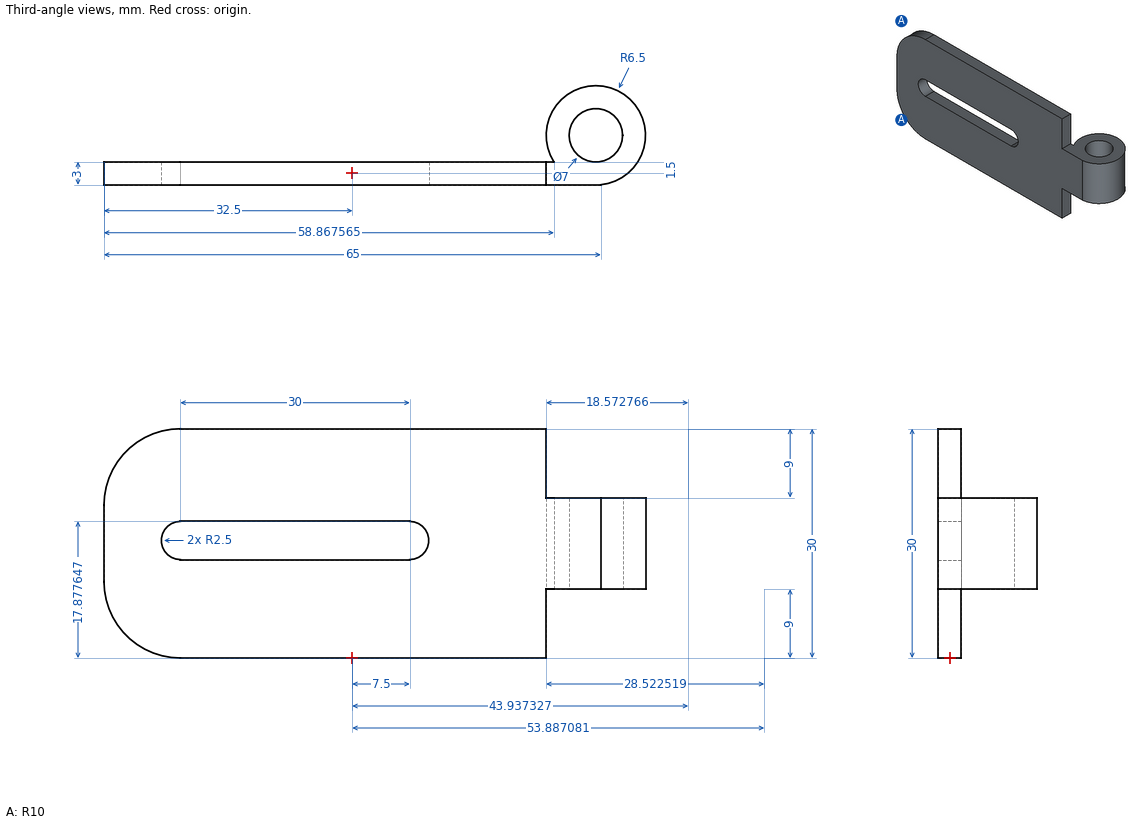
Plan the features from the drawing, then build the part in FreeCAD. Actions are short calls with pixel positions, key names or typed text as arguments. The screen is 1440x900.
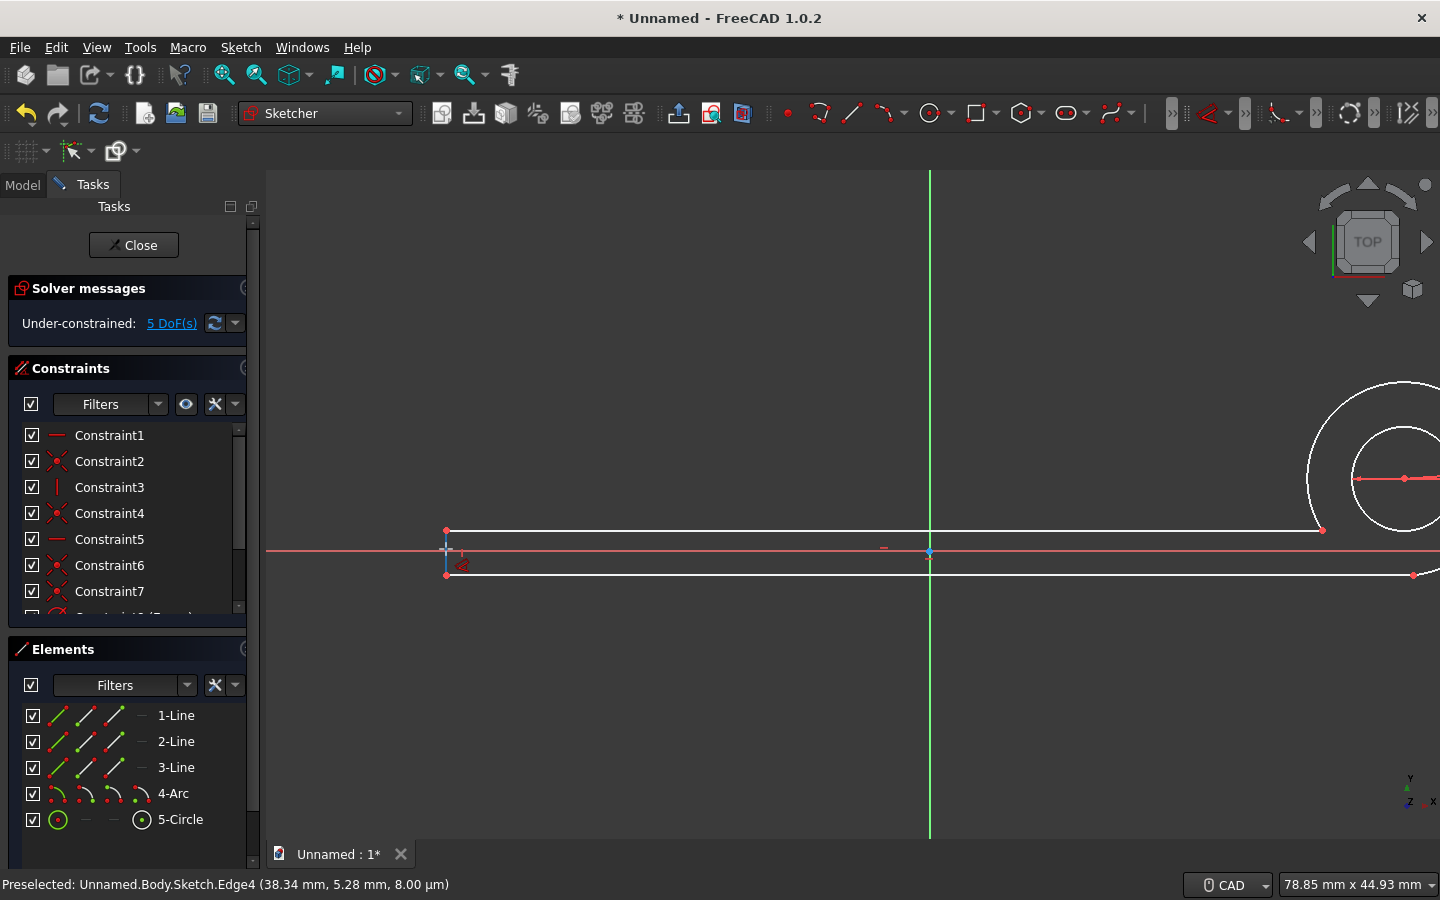
click(446, 549)
click(412, 537)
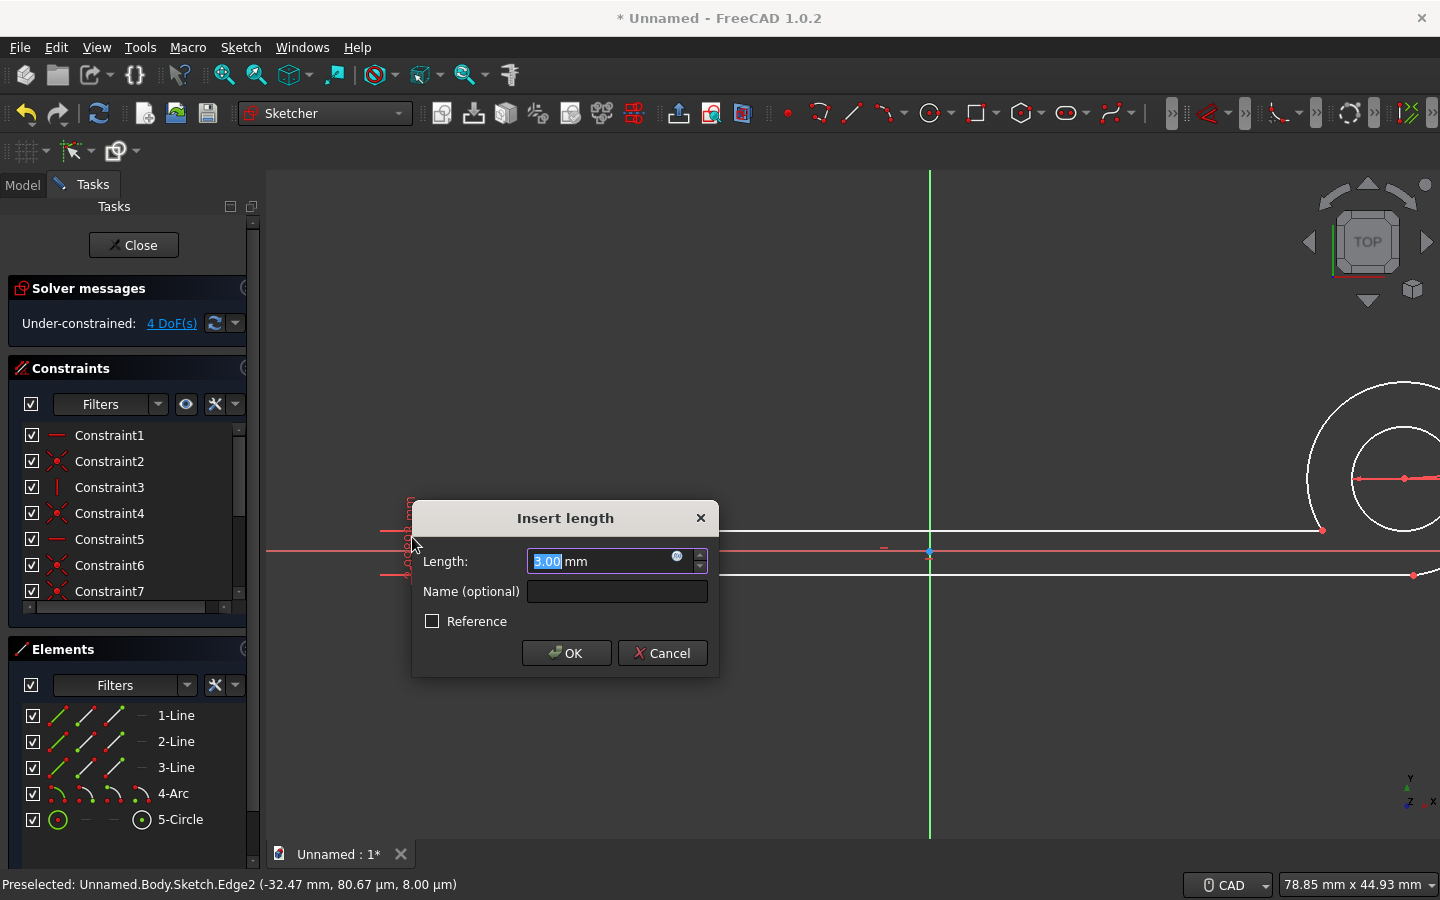
text(3)
key(Return)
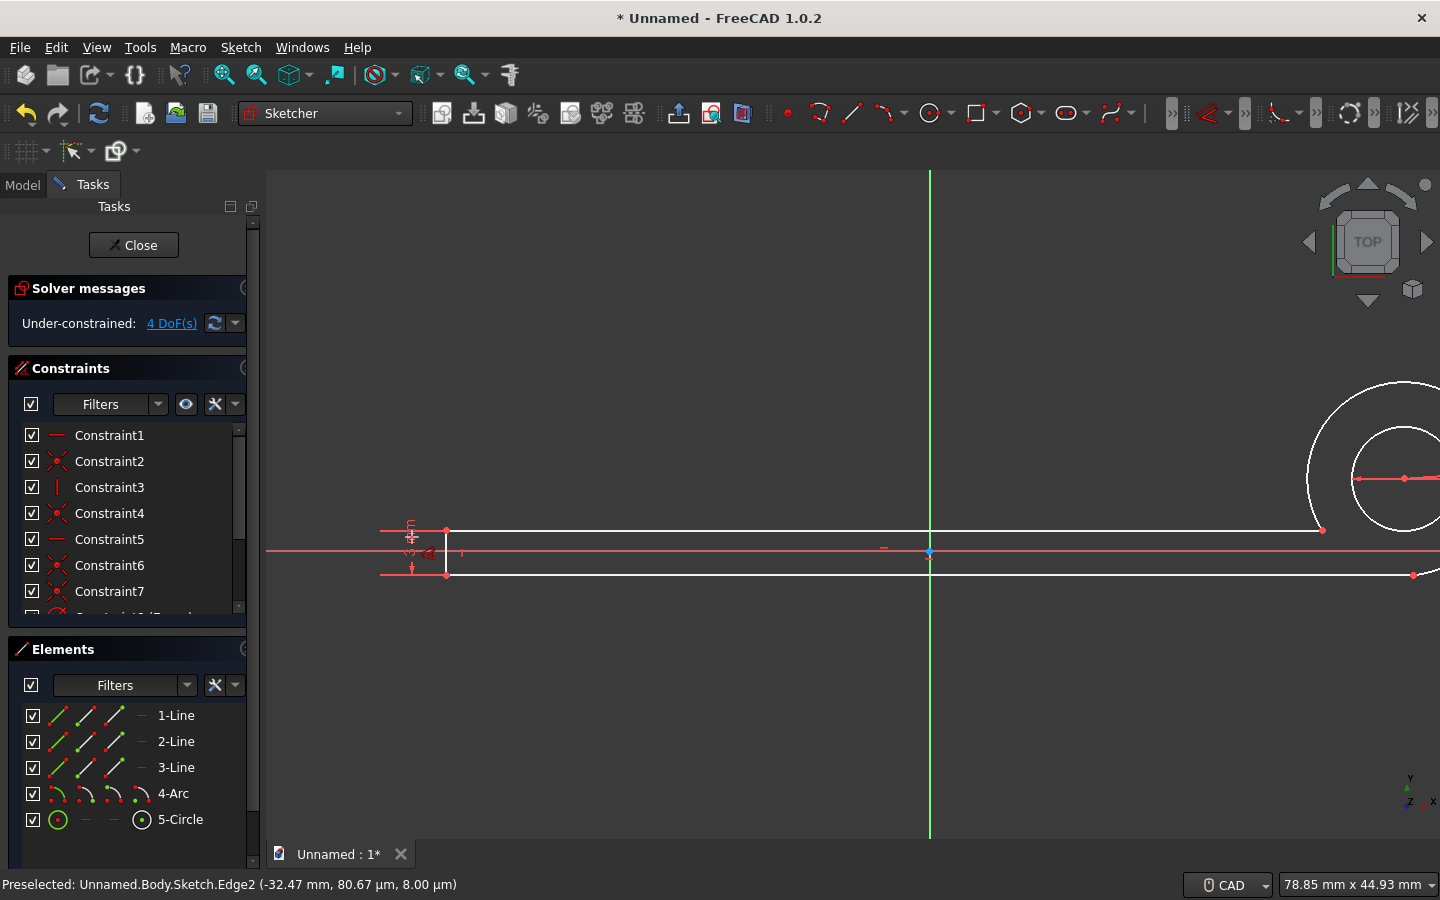
click(736, 575)
click(861, 609)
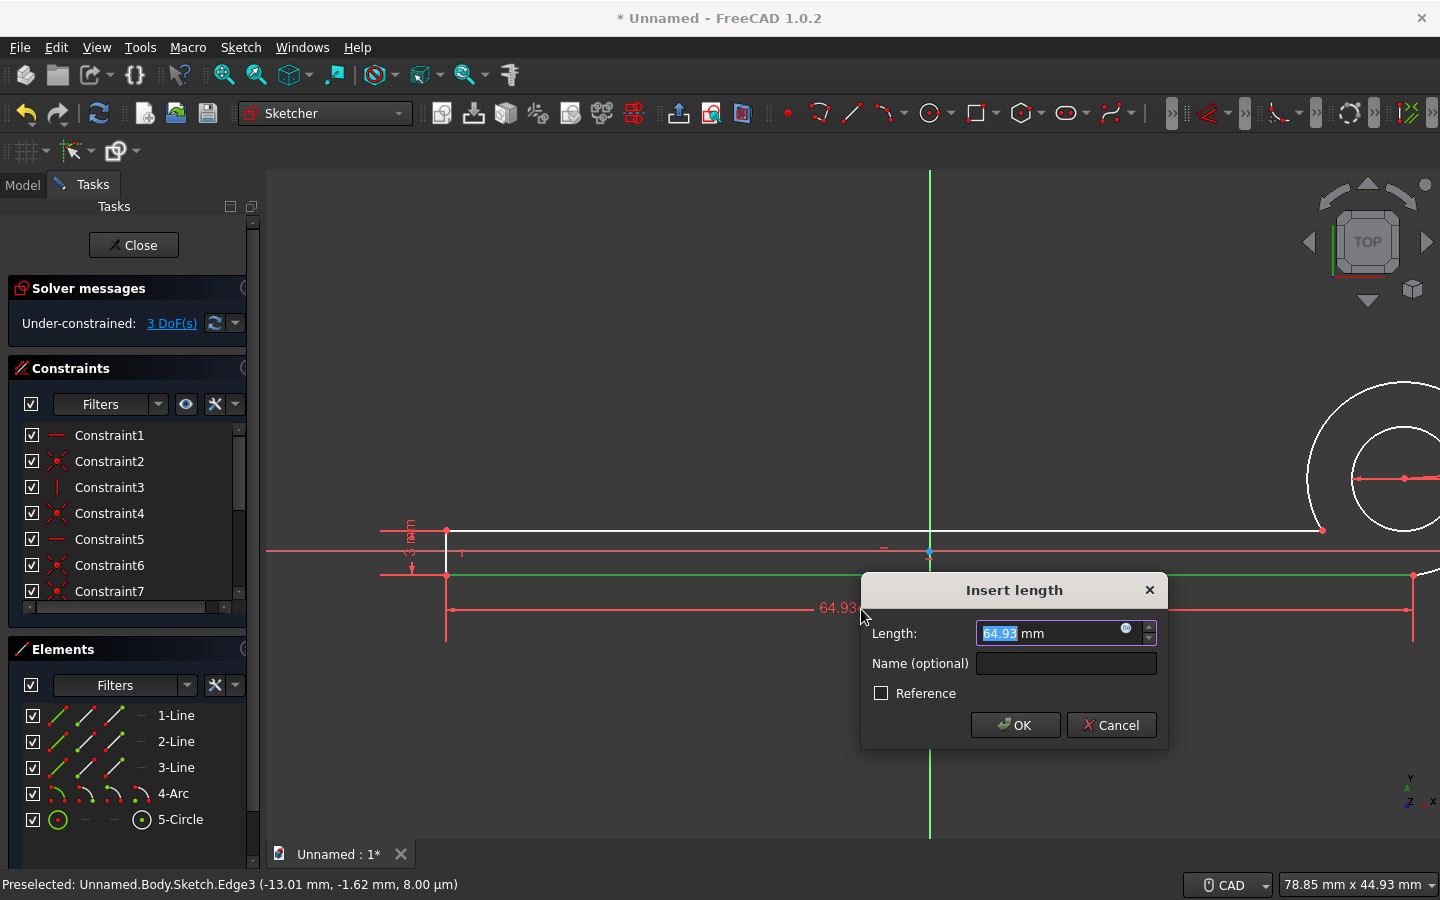
text(65)
key(Return)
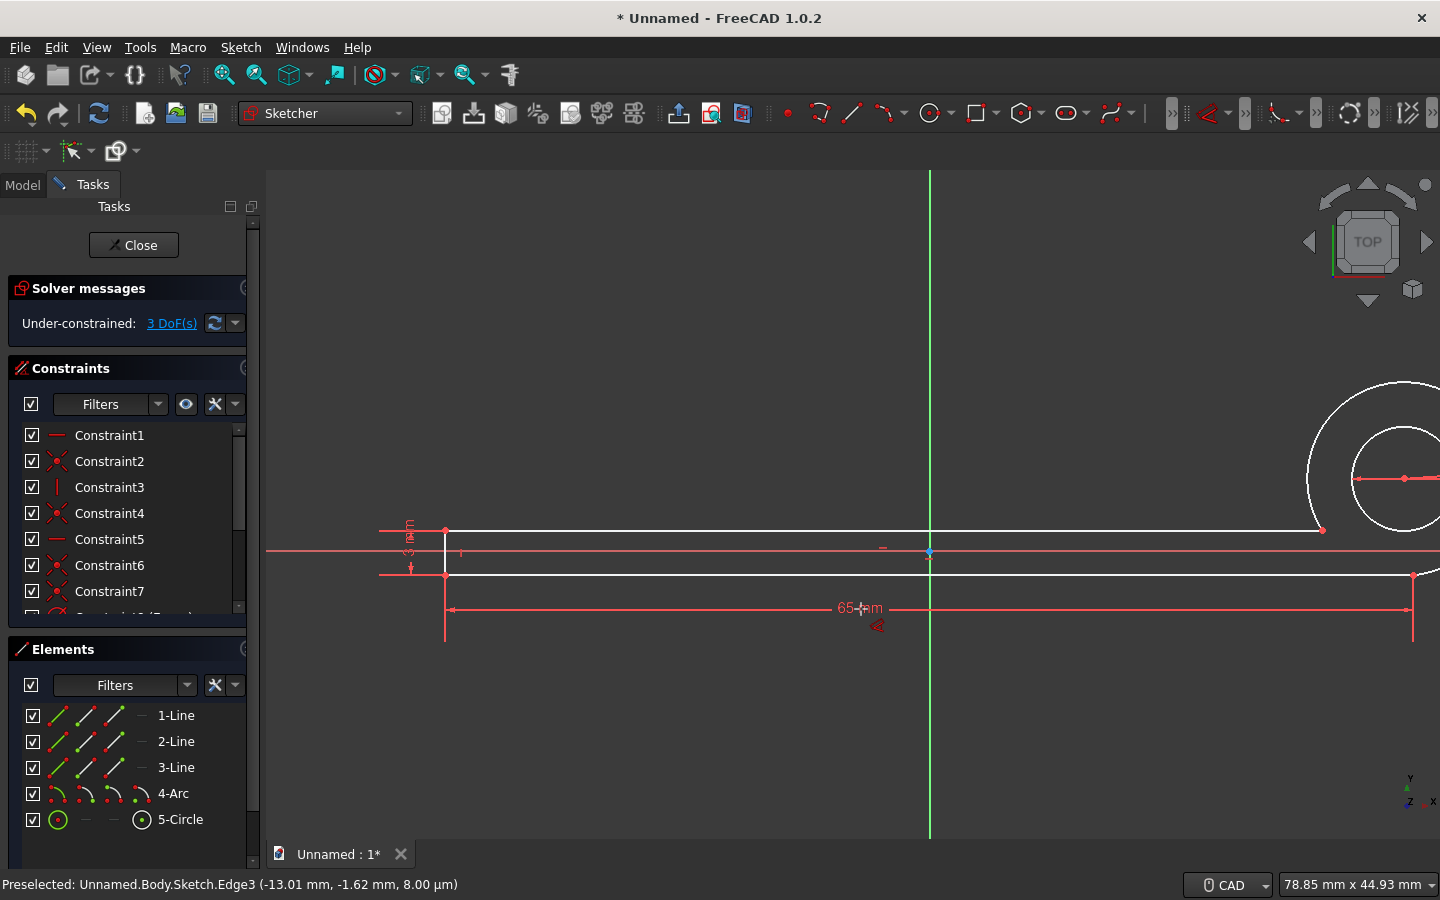
scroll(446, 550, down, 2)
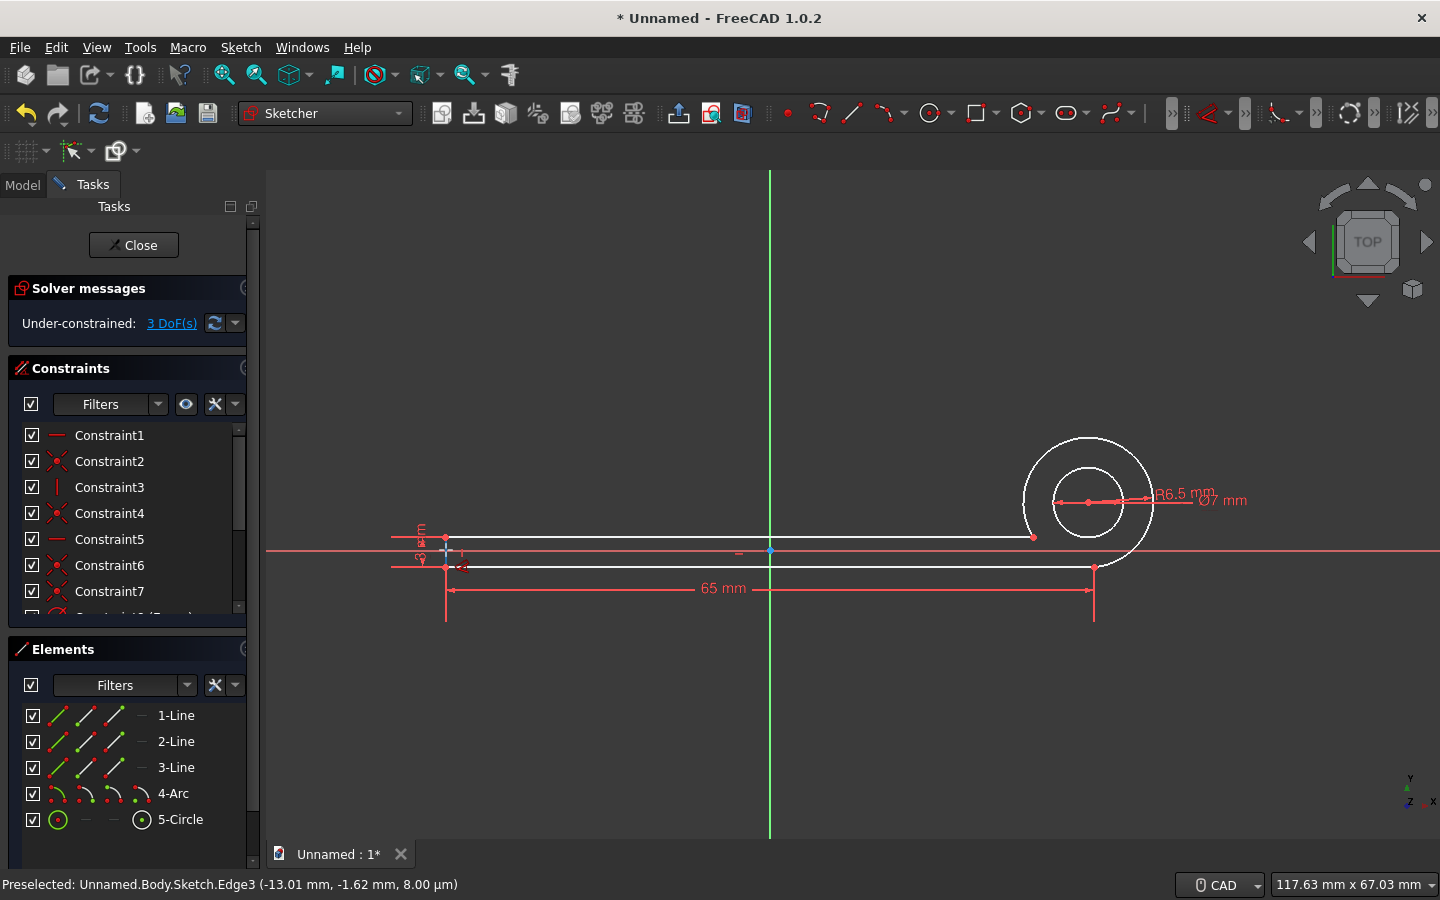
scroll(1033, 537, up, 5)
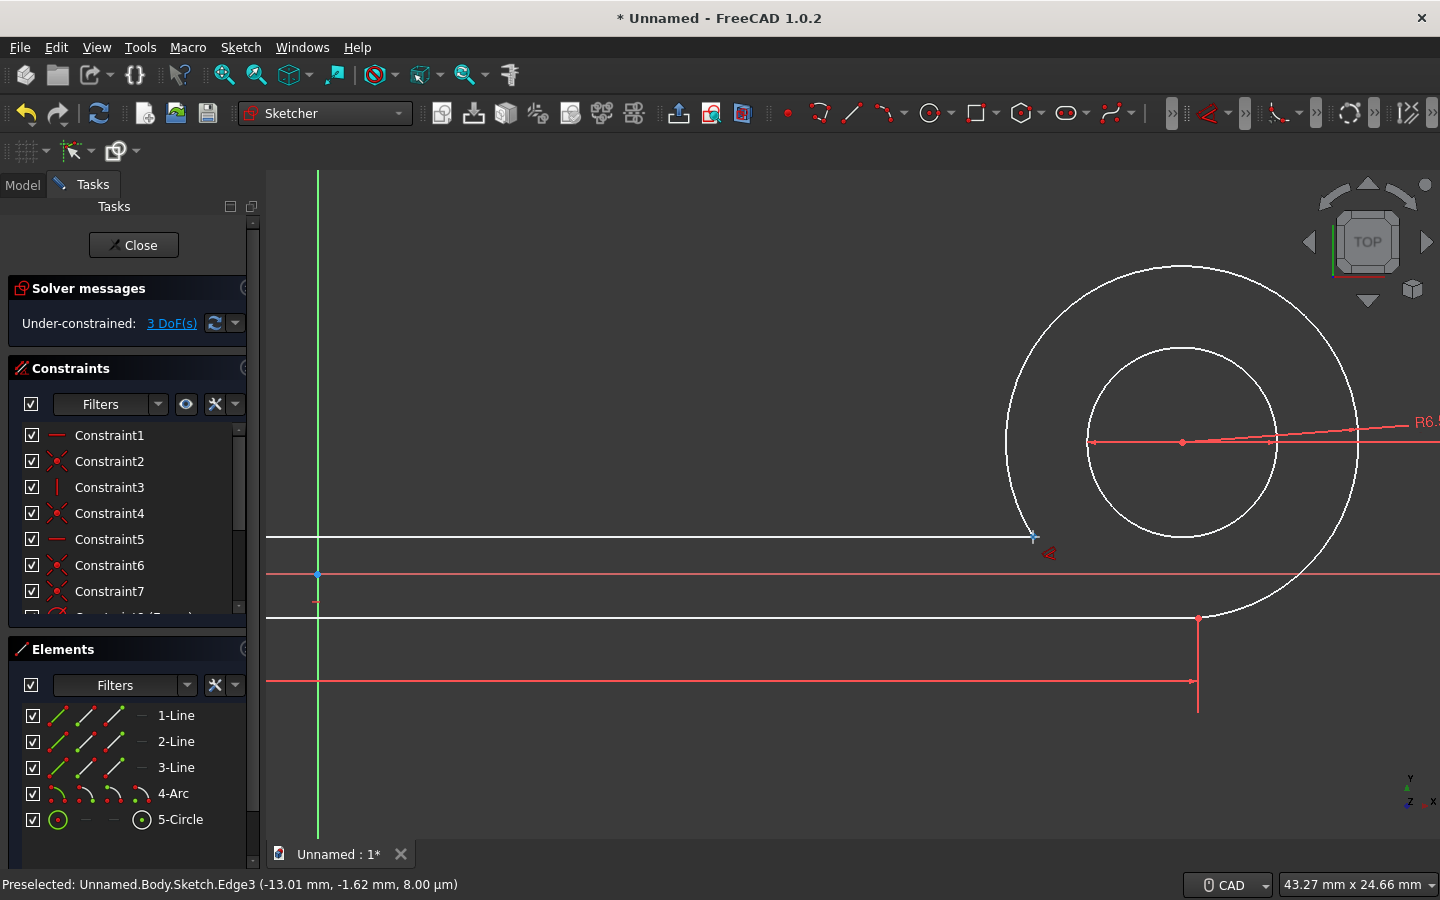
click(1033, 537)
click(1067, 555)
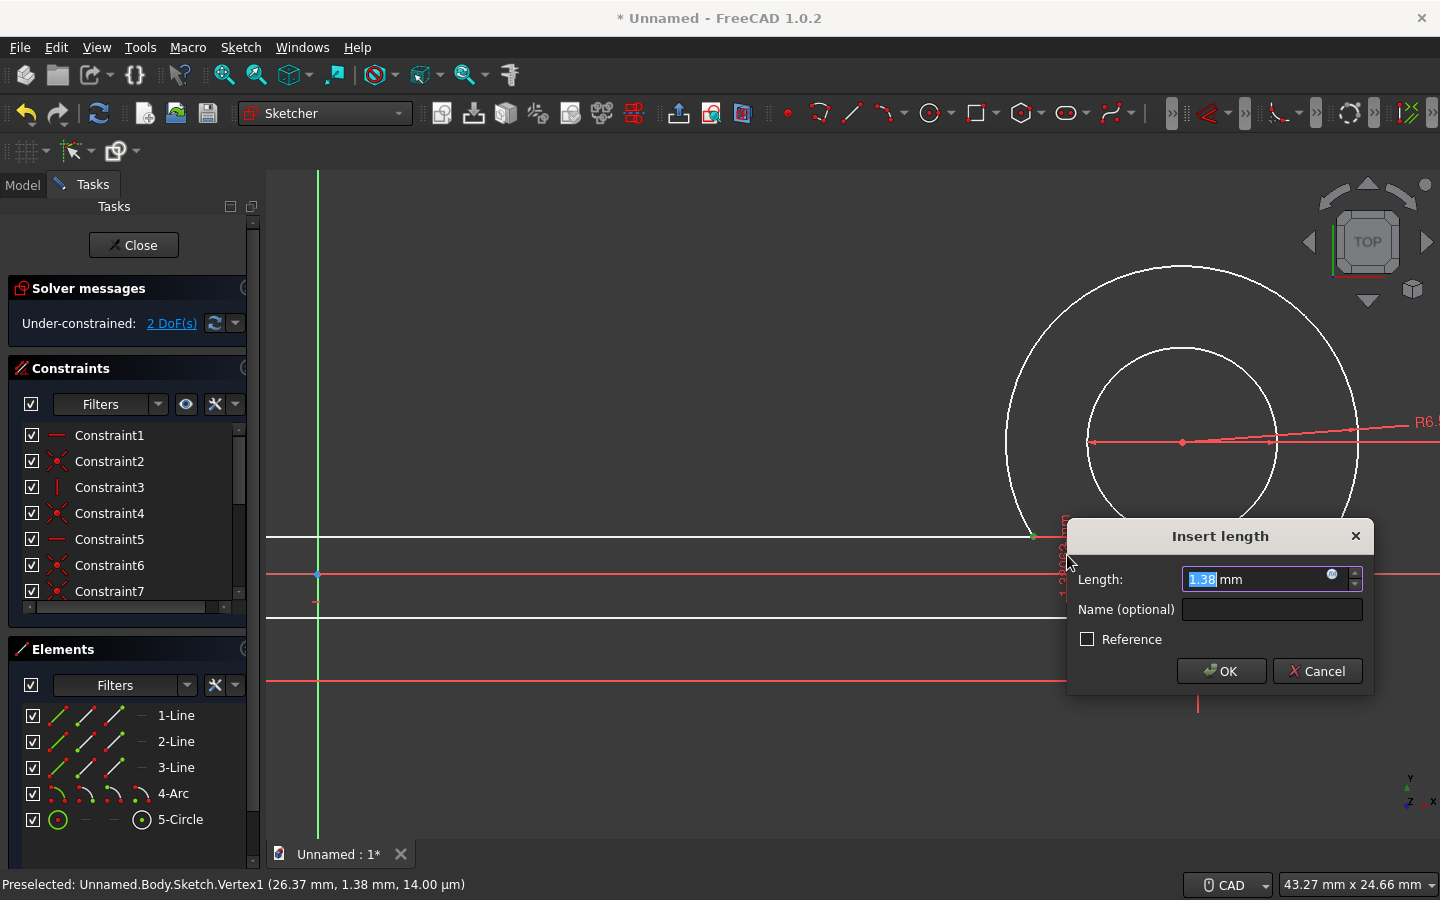
text(1.5)
key(Return)